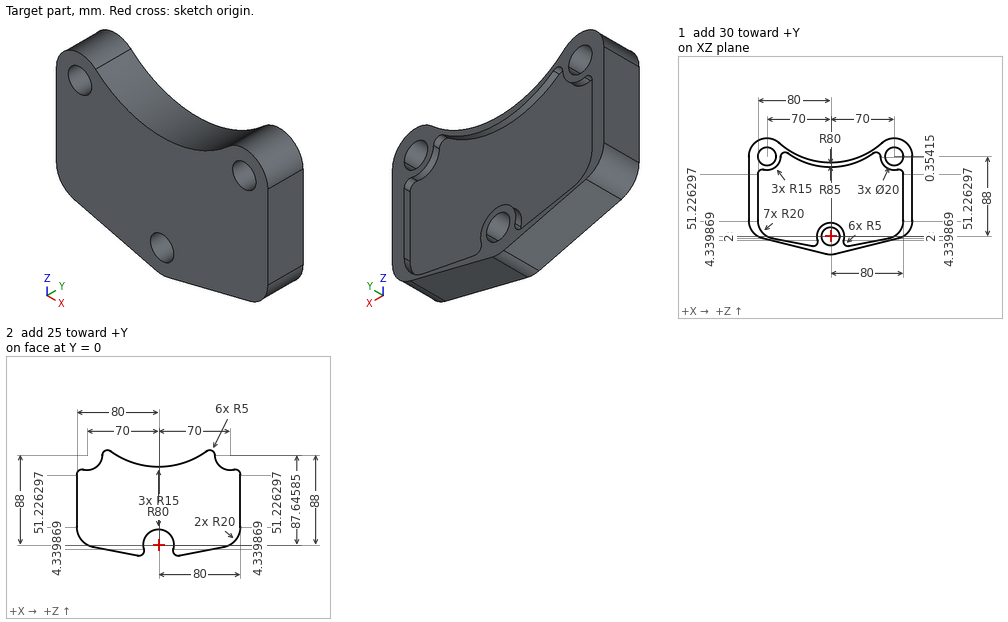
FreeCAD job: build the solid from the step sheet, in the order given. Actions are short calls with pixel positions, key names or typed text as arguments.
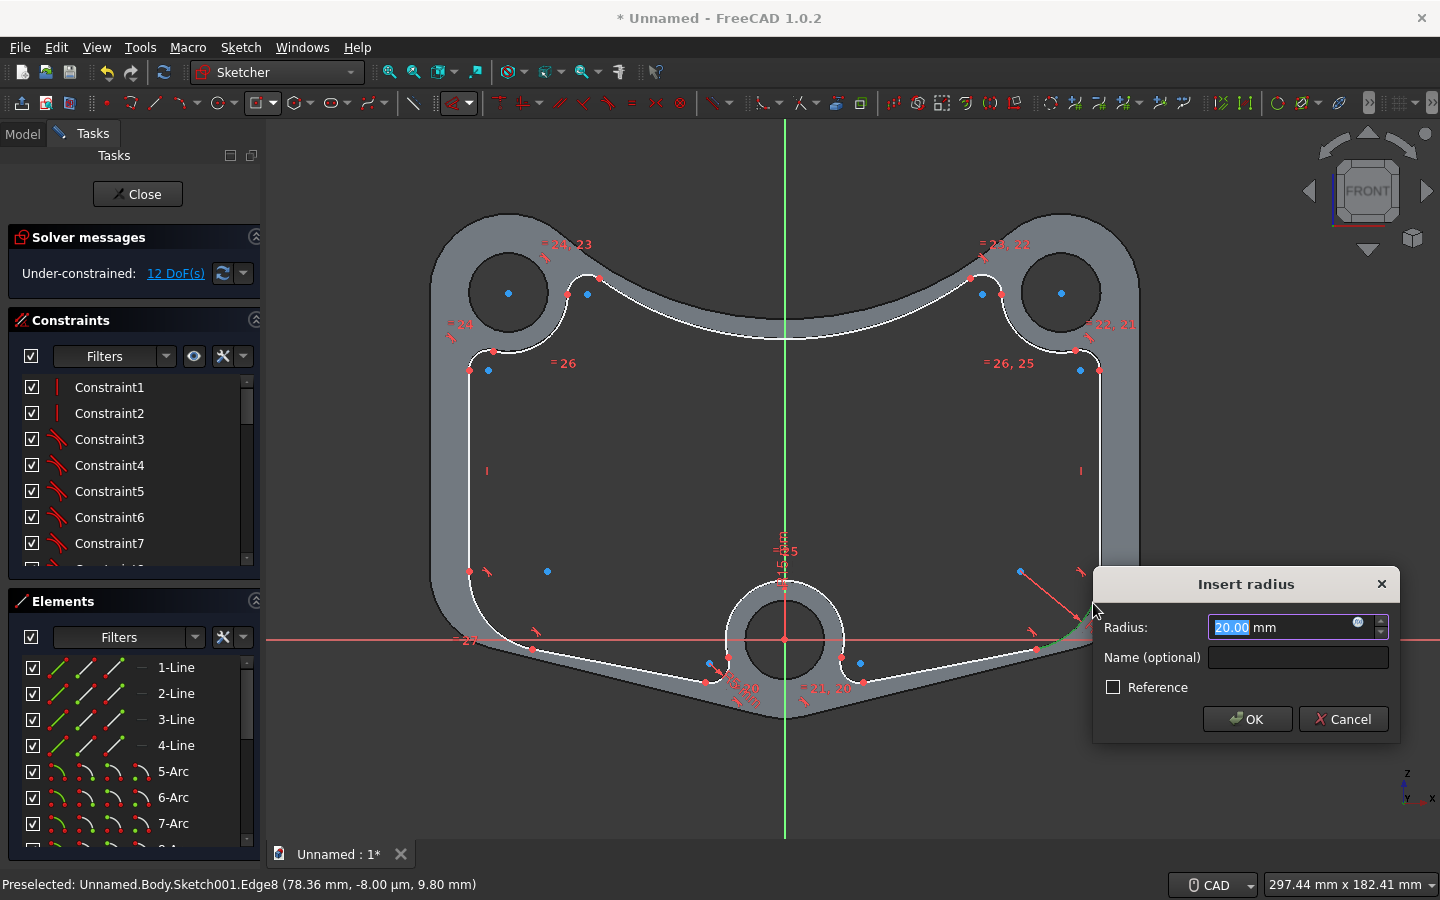
text(20)
key(Return)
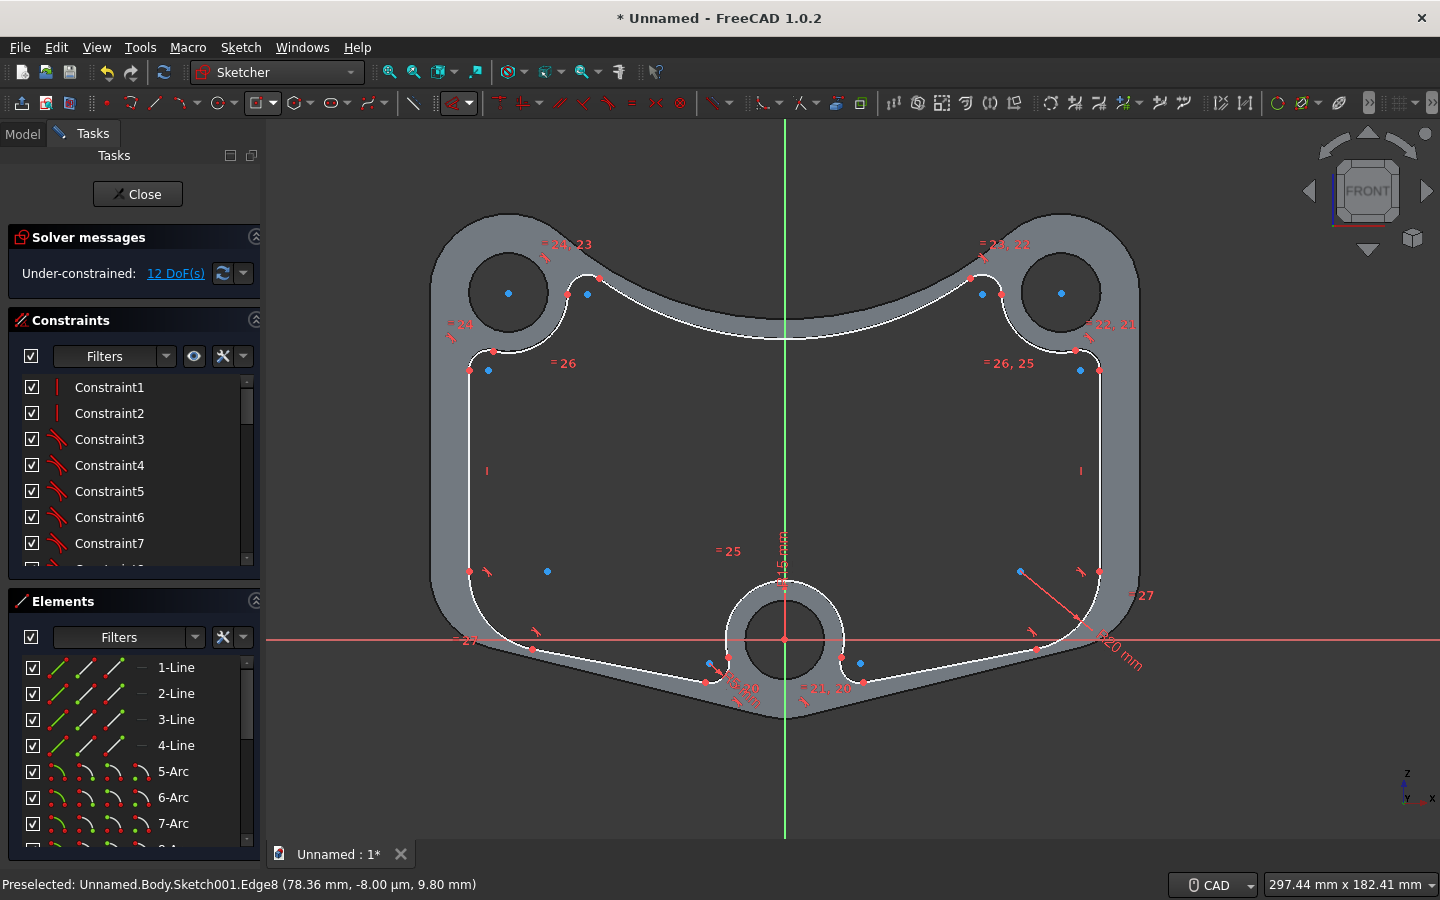
click(706, 329)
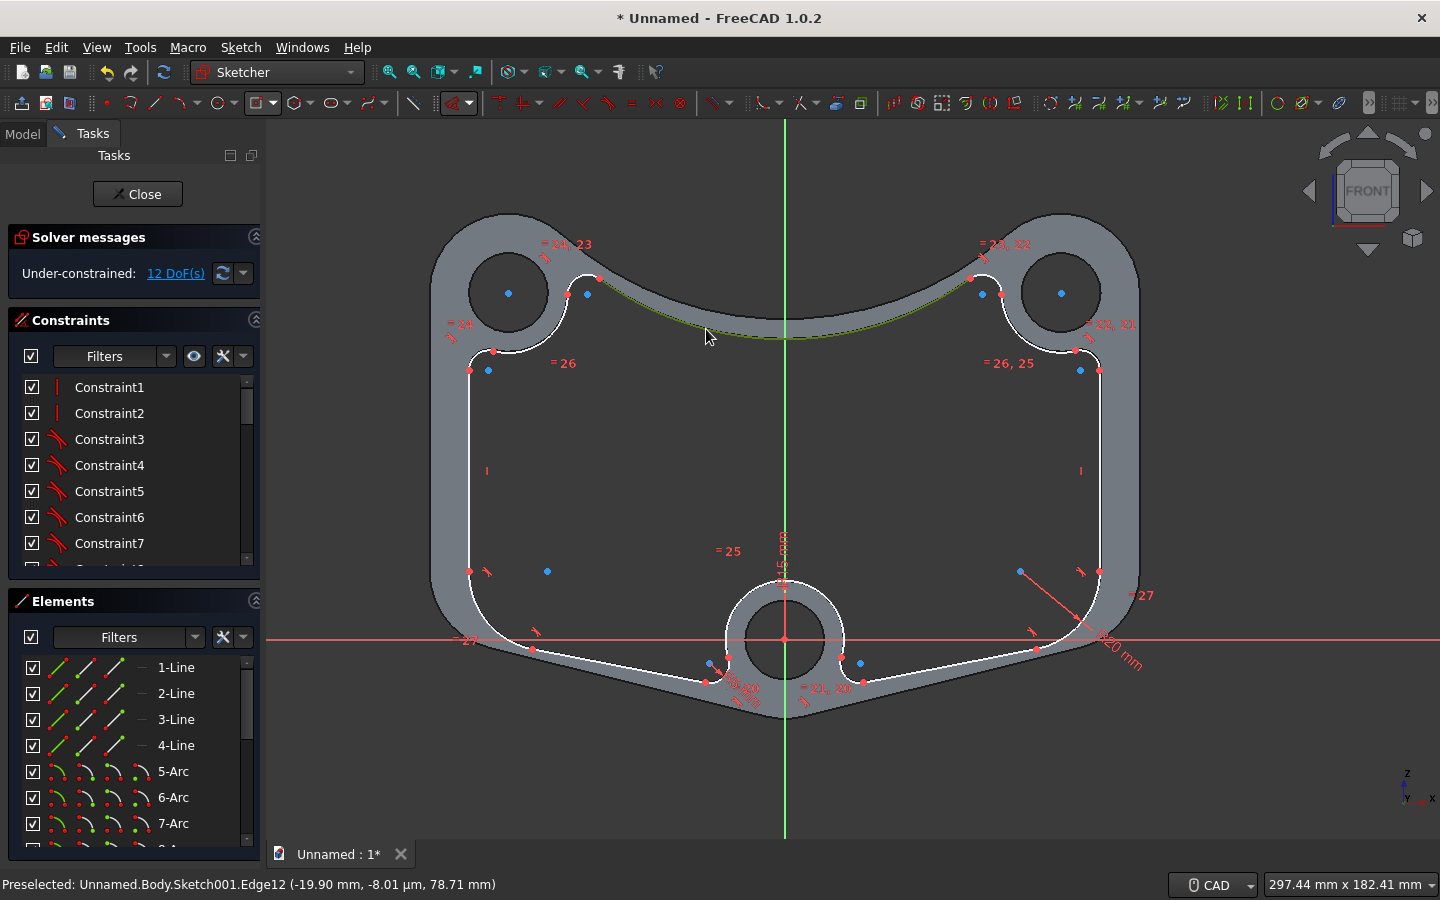
key(k)
key(r)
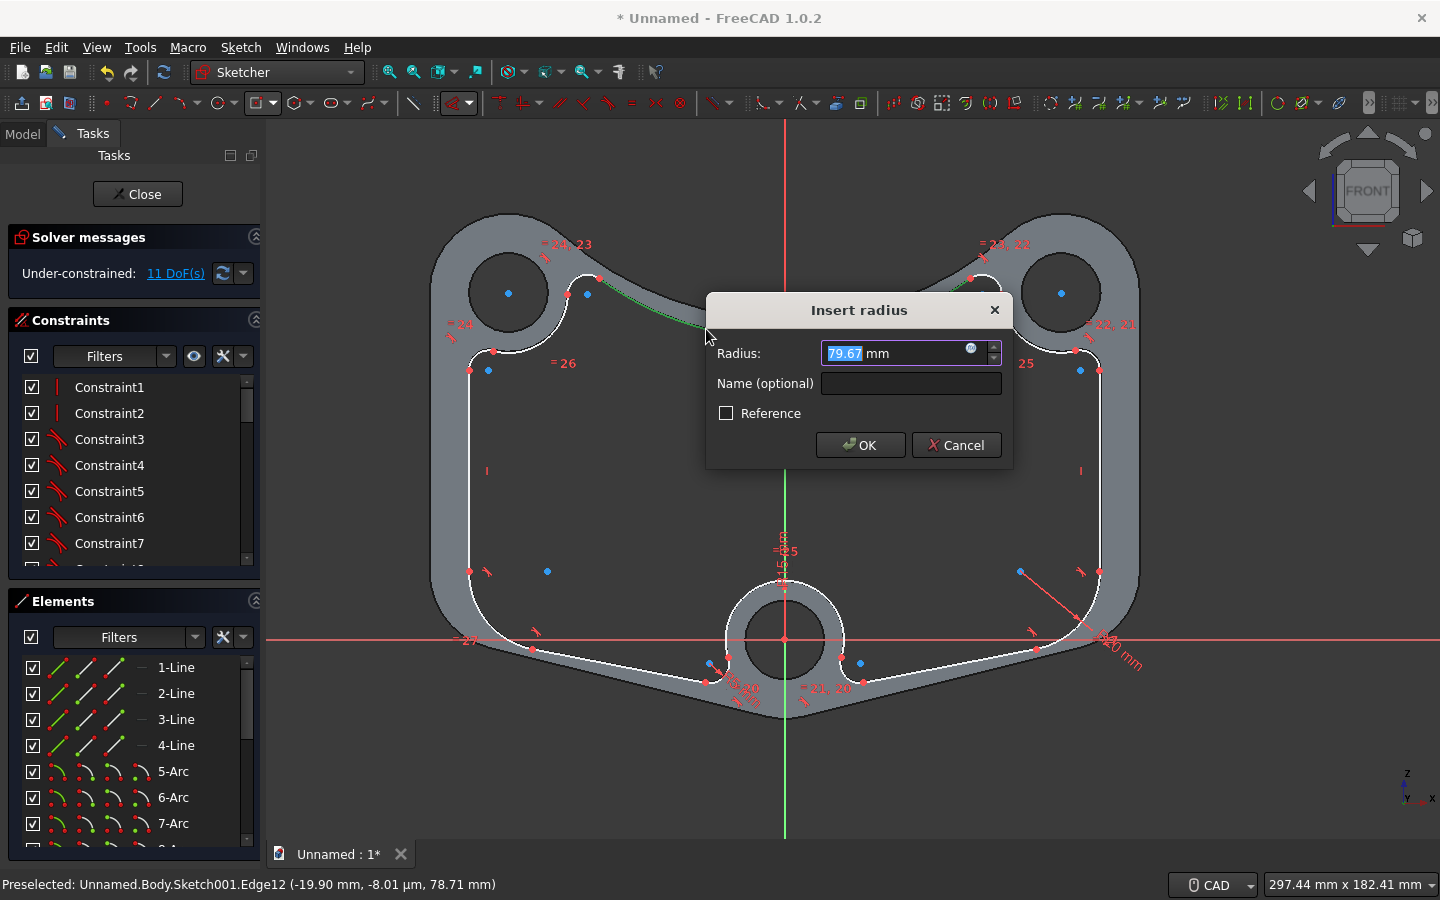
text(80)
key(Return)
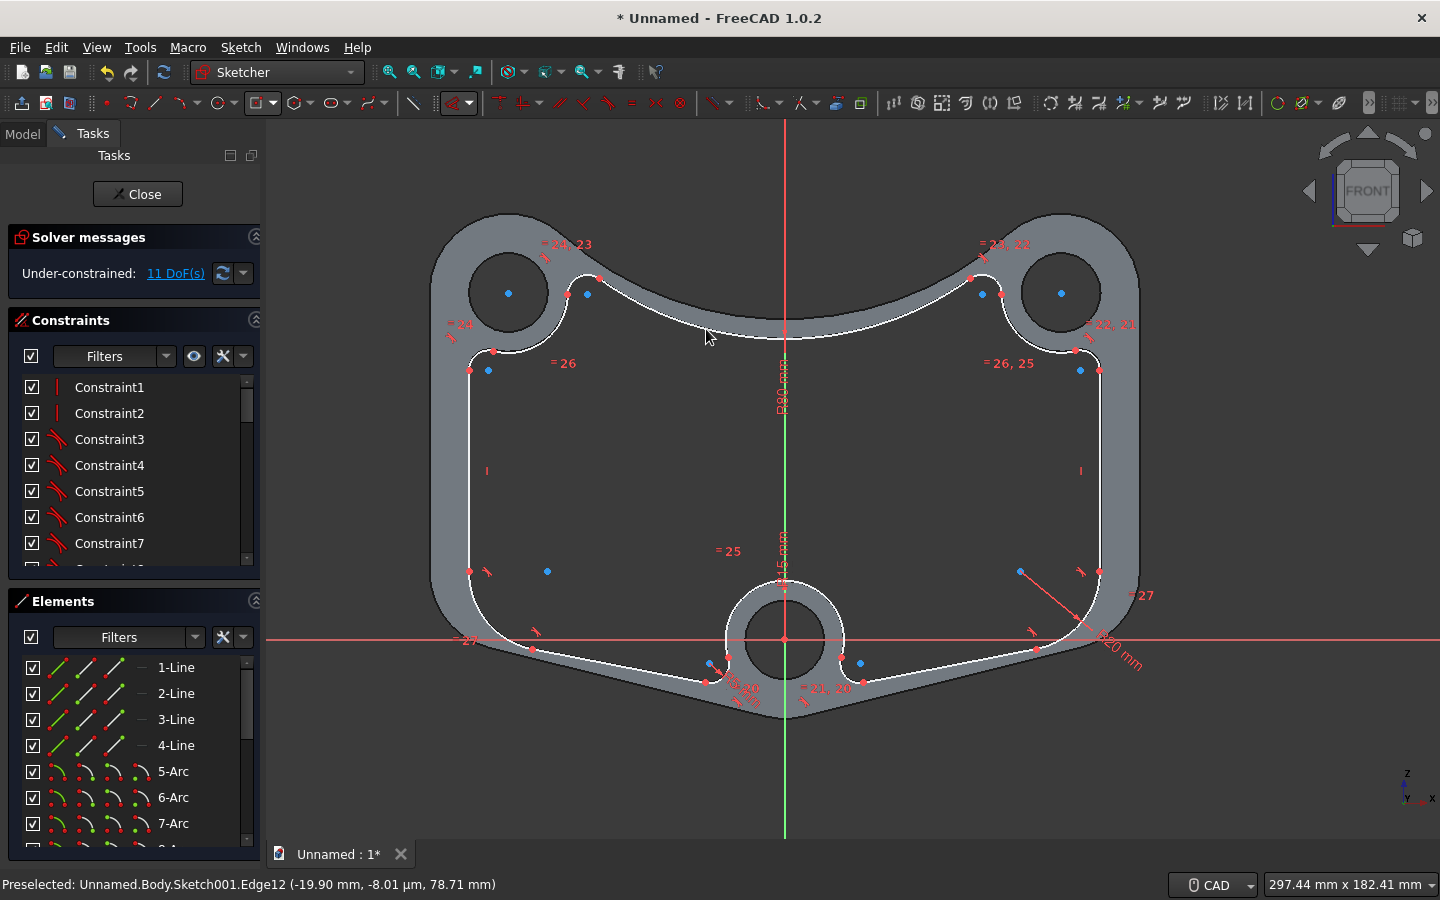
click(1100, 572)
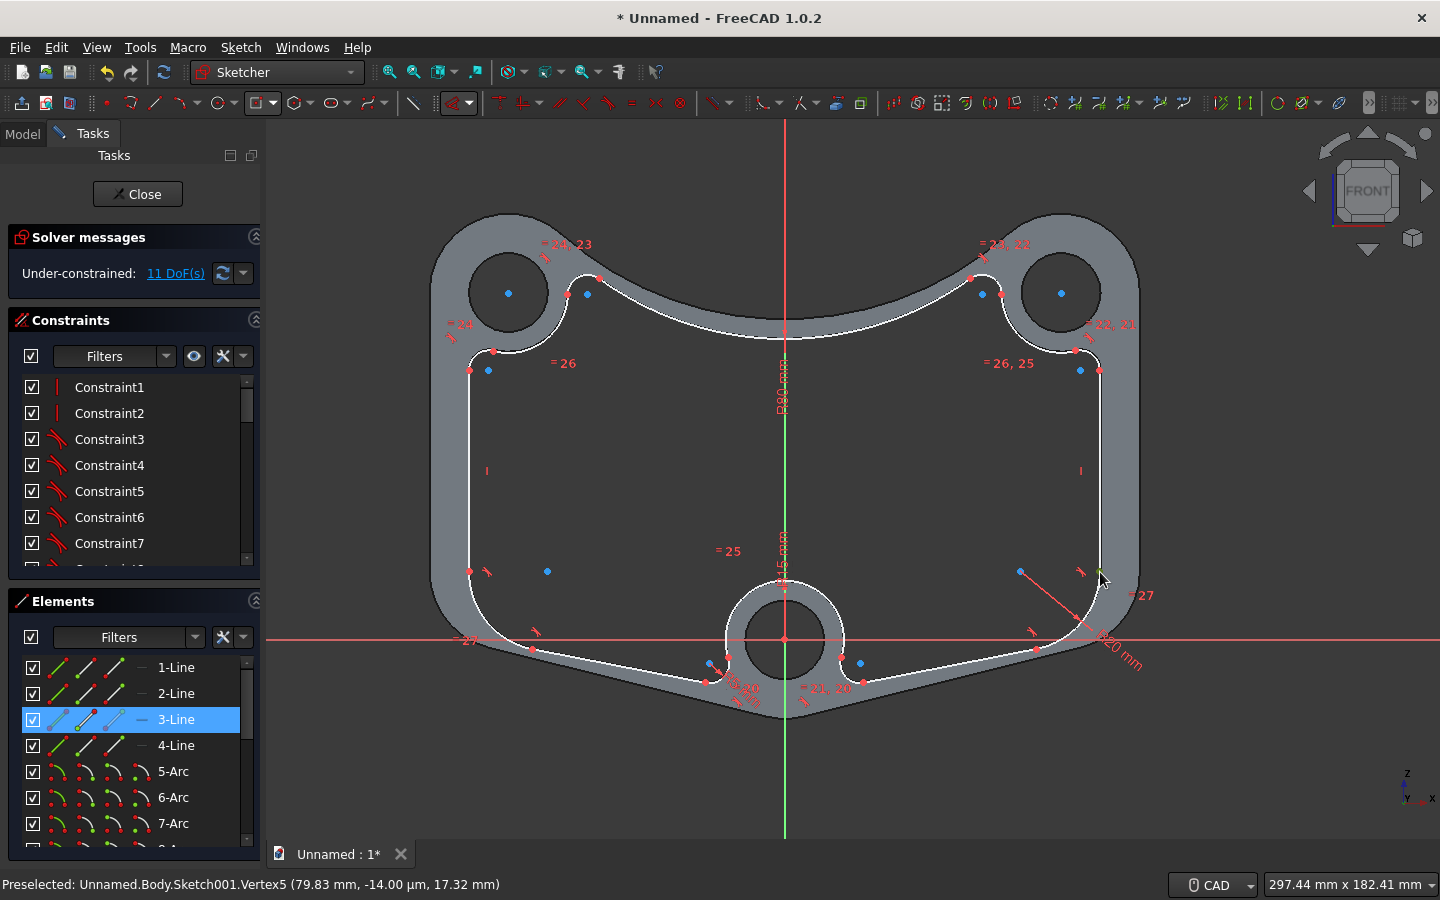
key(l)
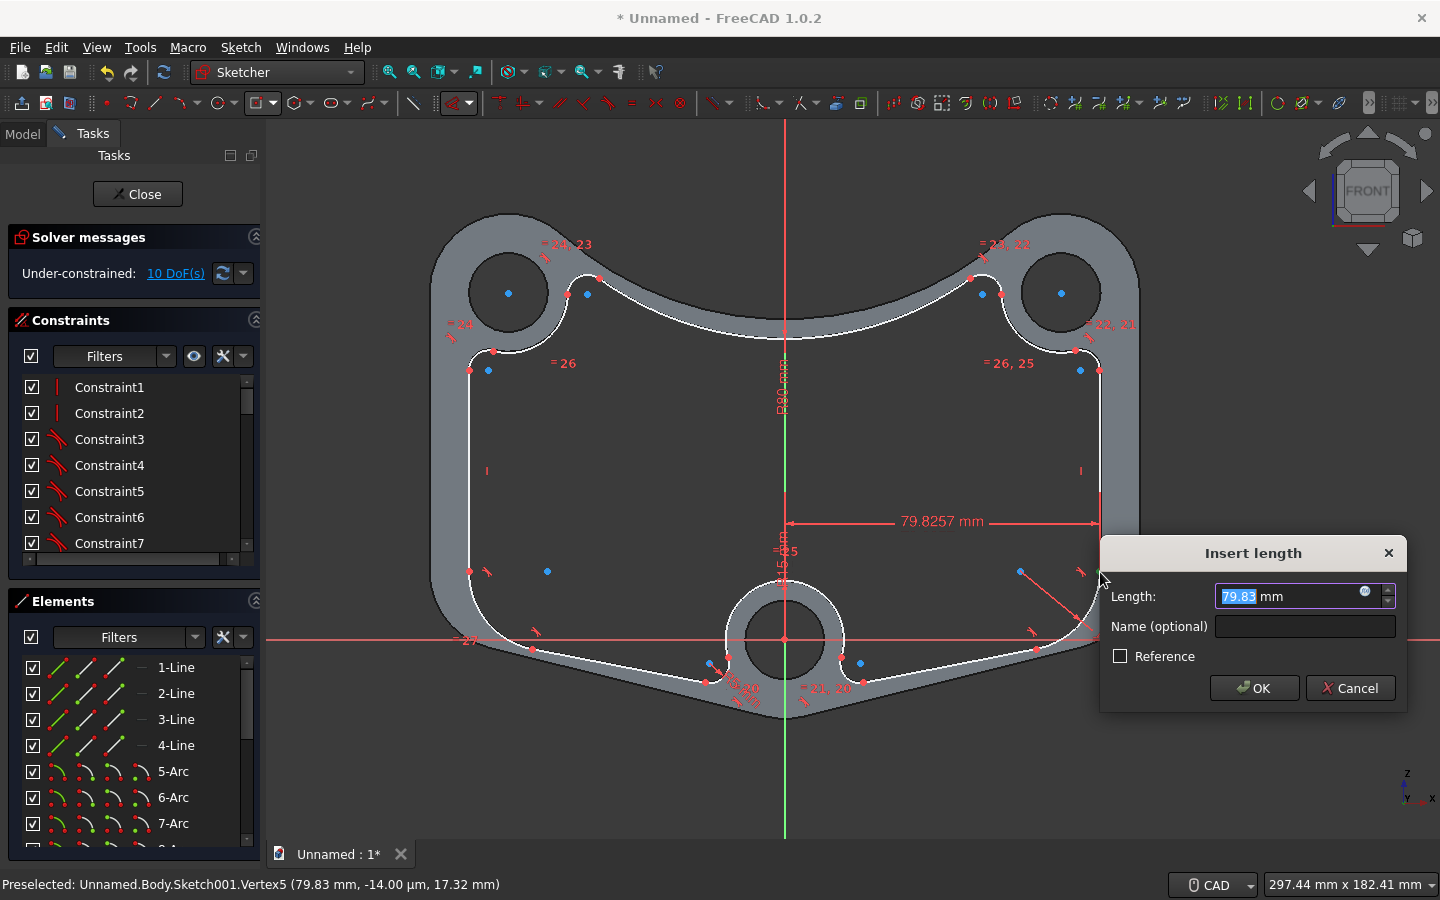
text(80)
key(Return)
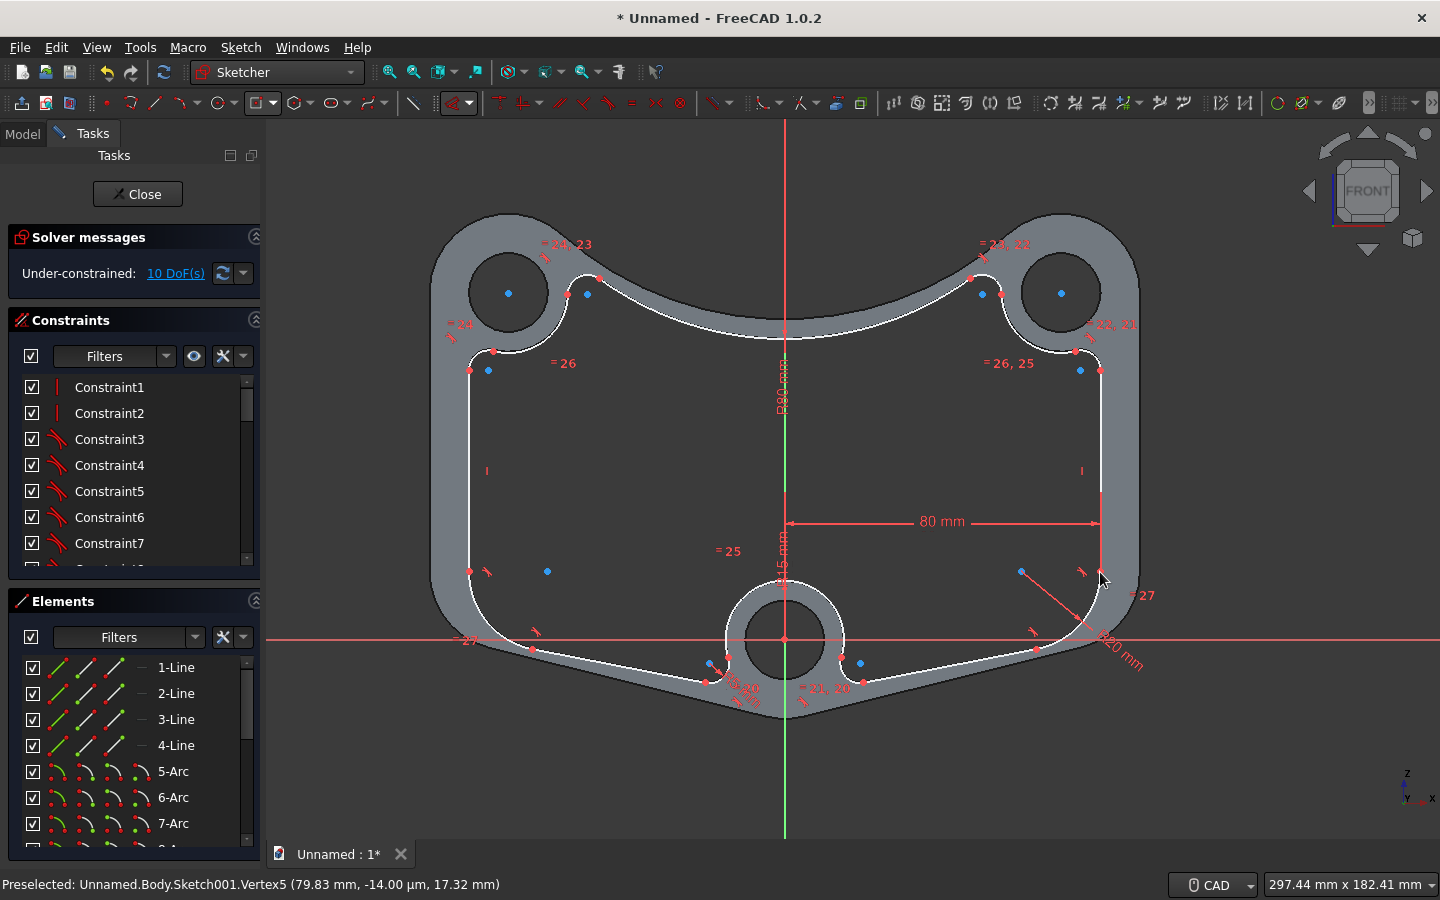
click(469, 370)